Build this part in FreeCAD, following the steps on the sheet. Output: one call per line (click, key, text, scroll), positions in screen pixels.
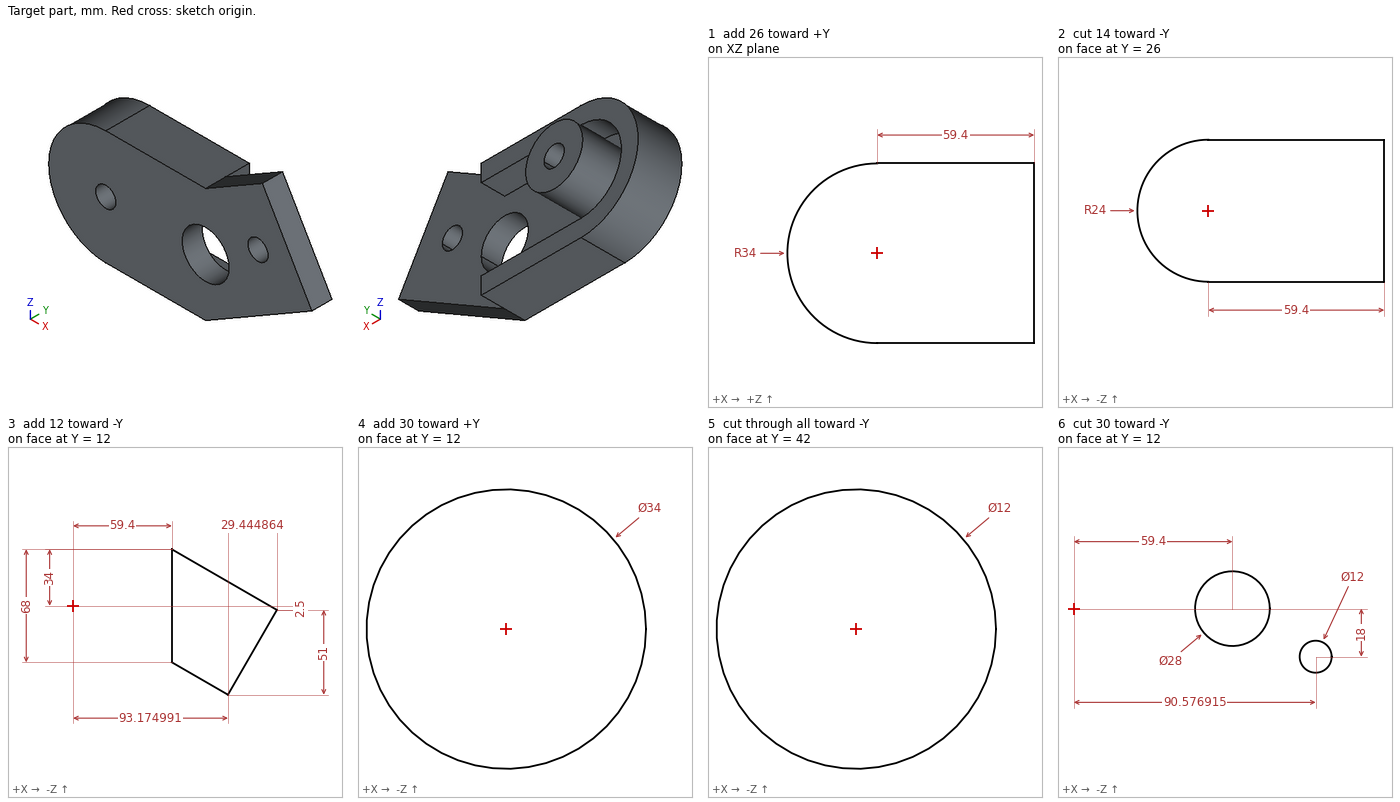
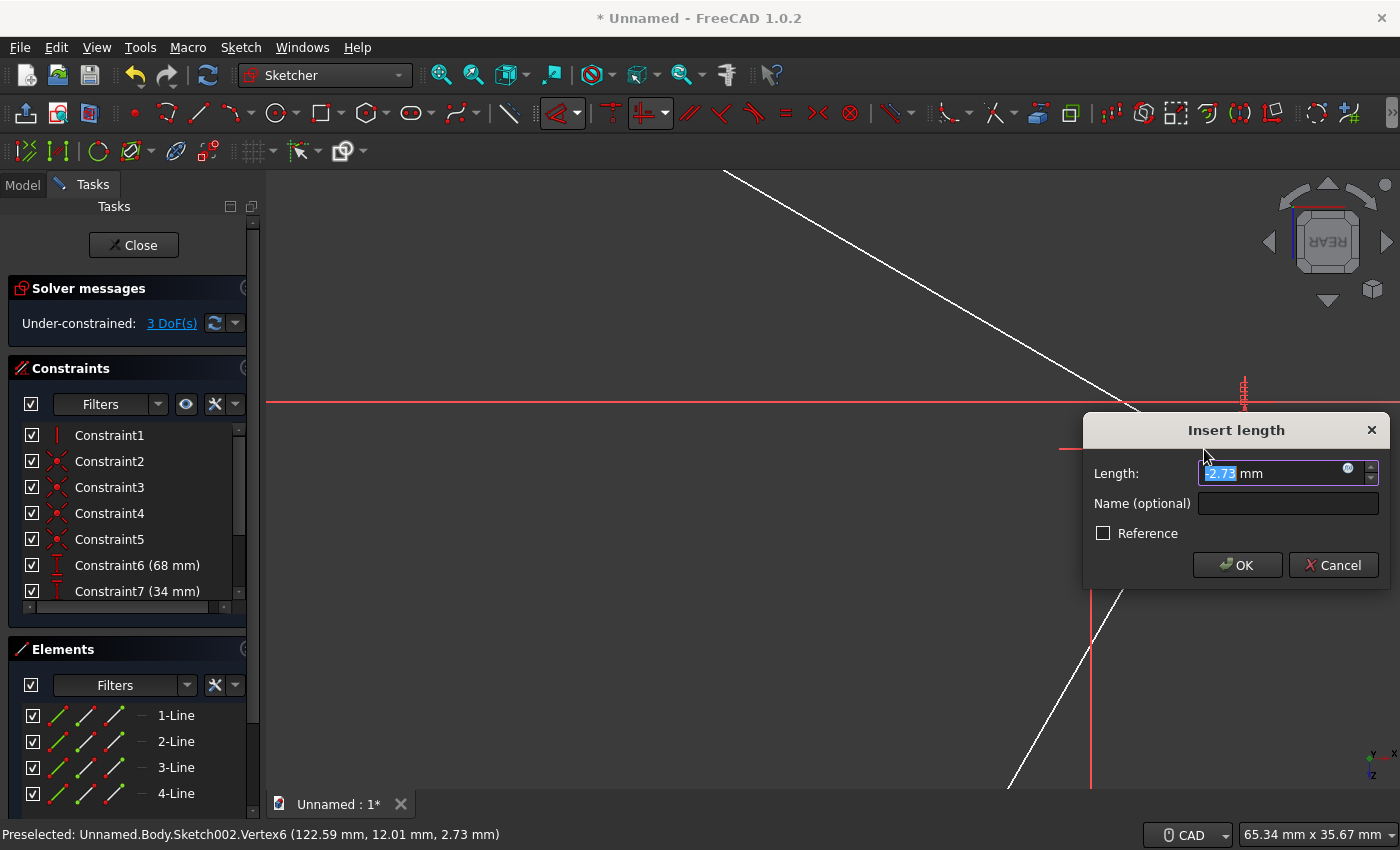
text(-2.5)
key(Return)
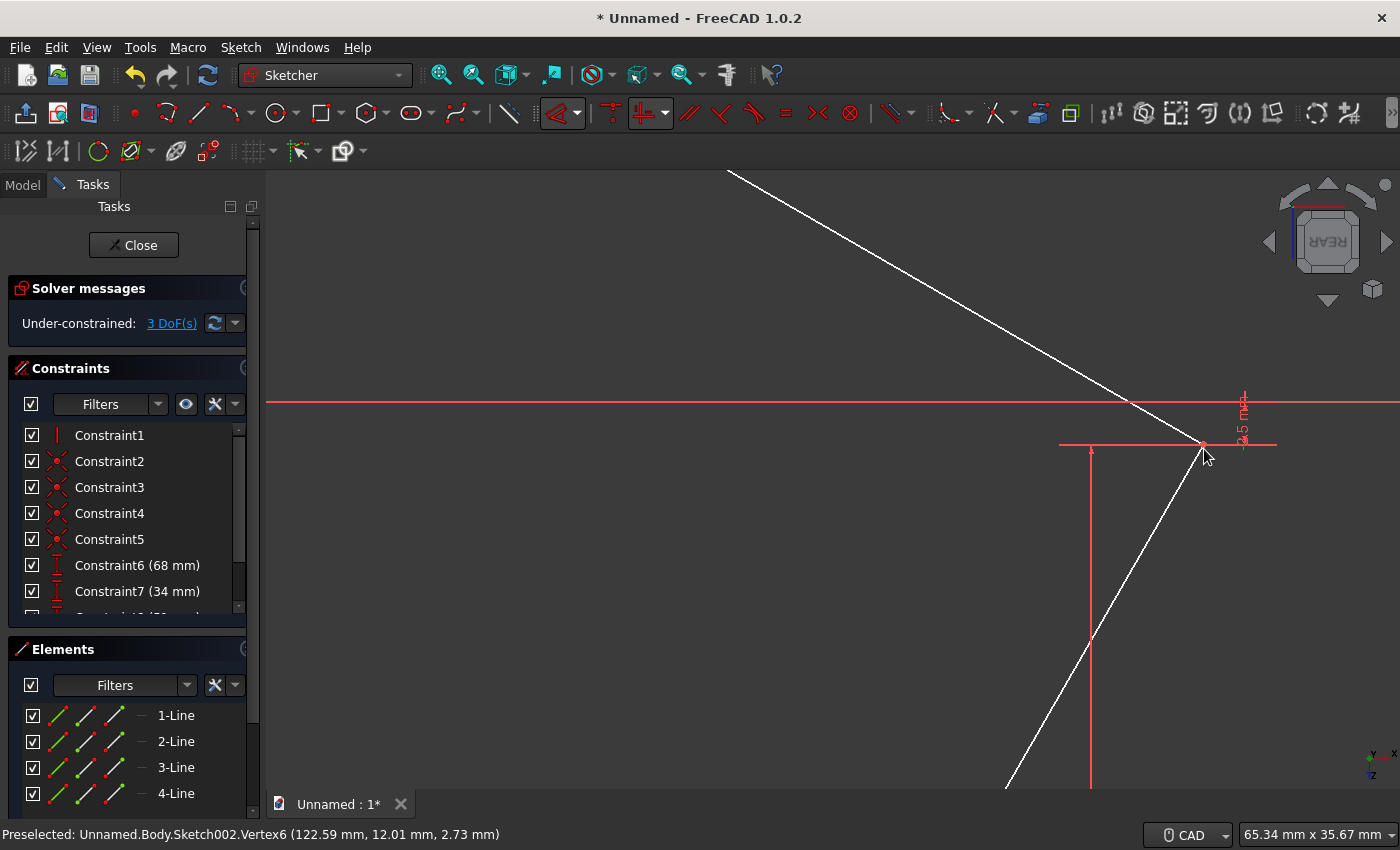
scroll(969, 450, down, 7)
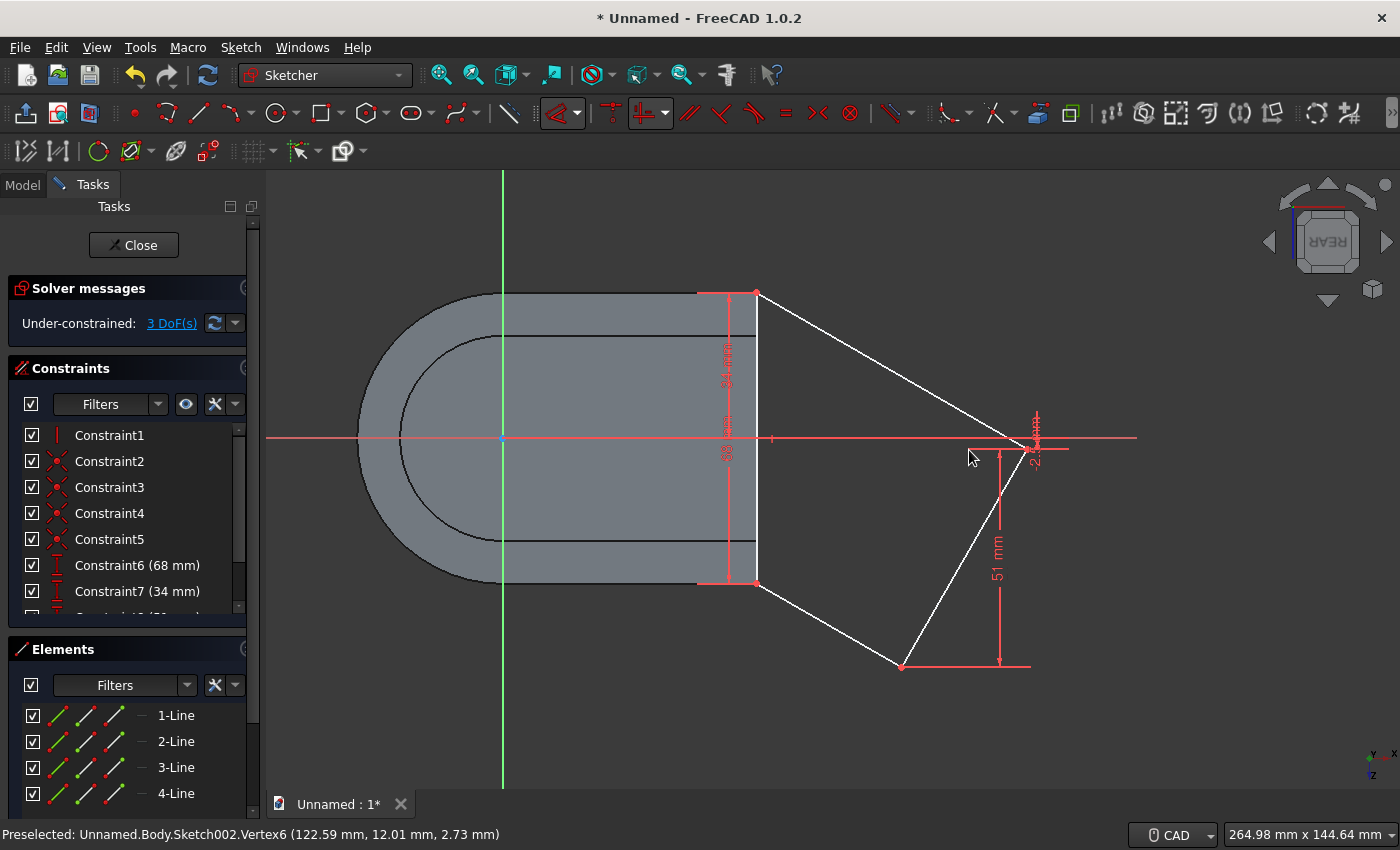
click(757, 293)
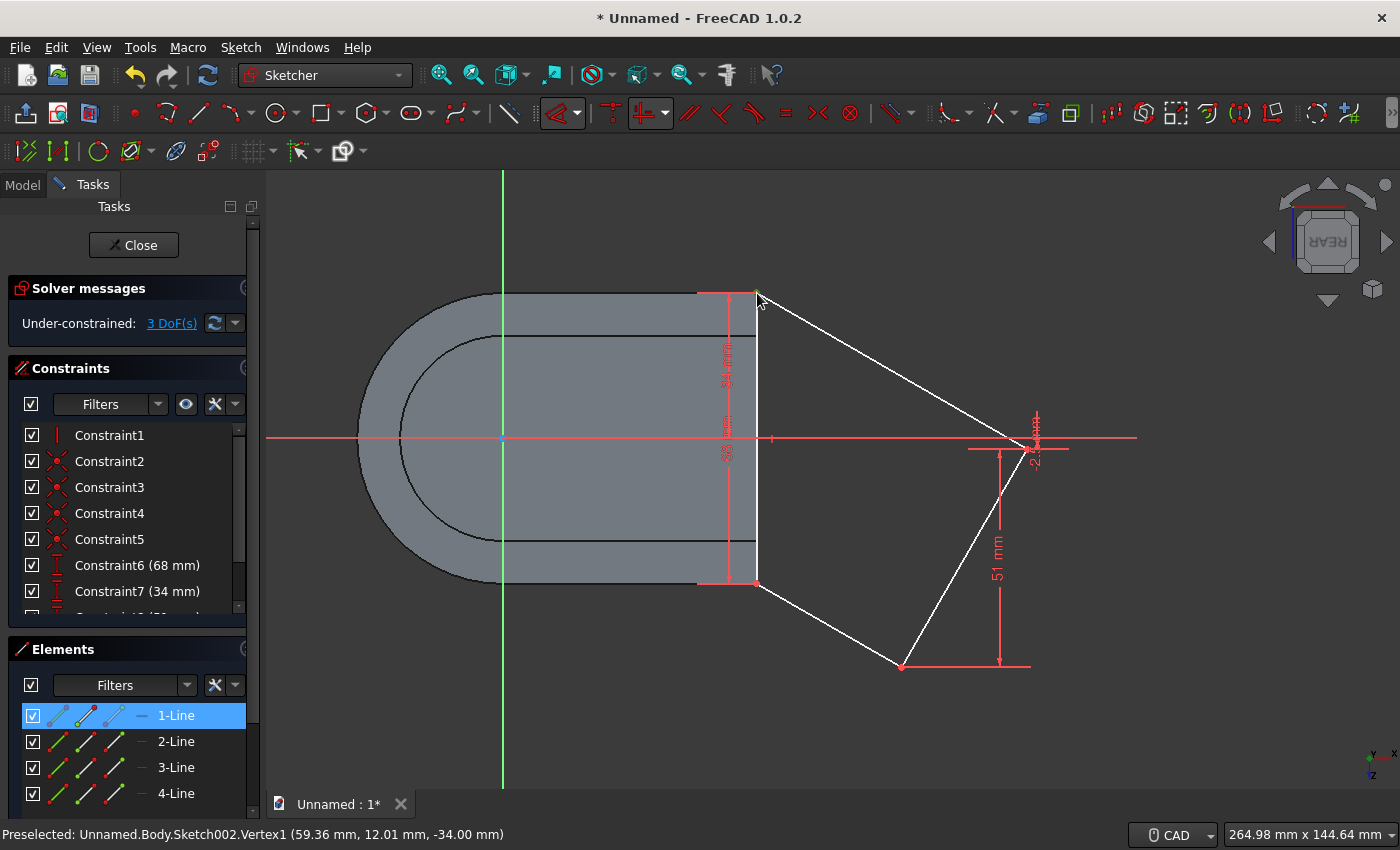
key(l)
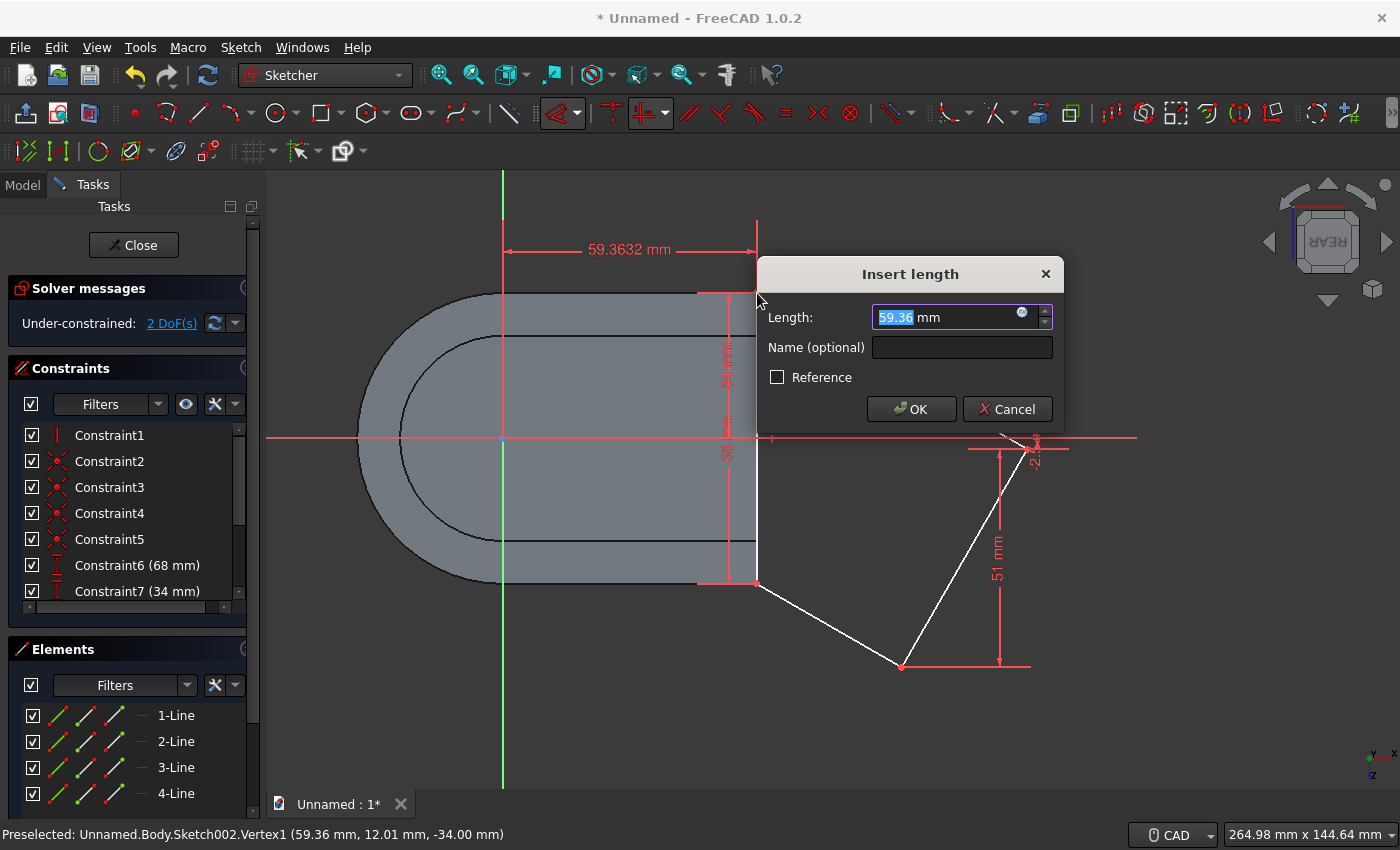
text(59.4)
key(Return)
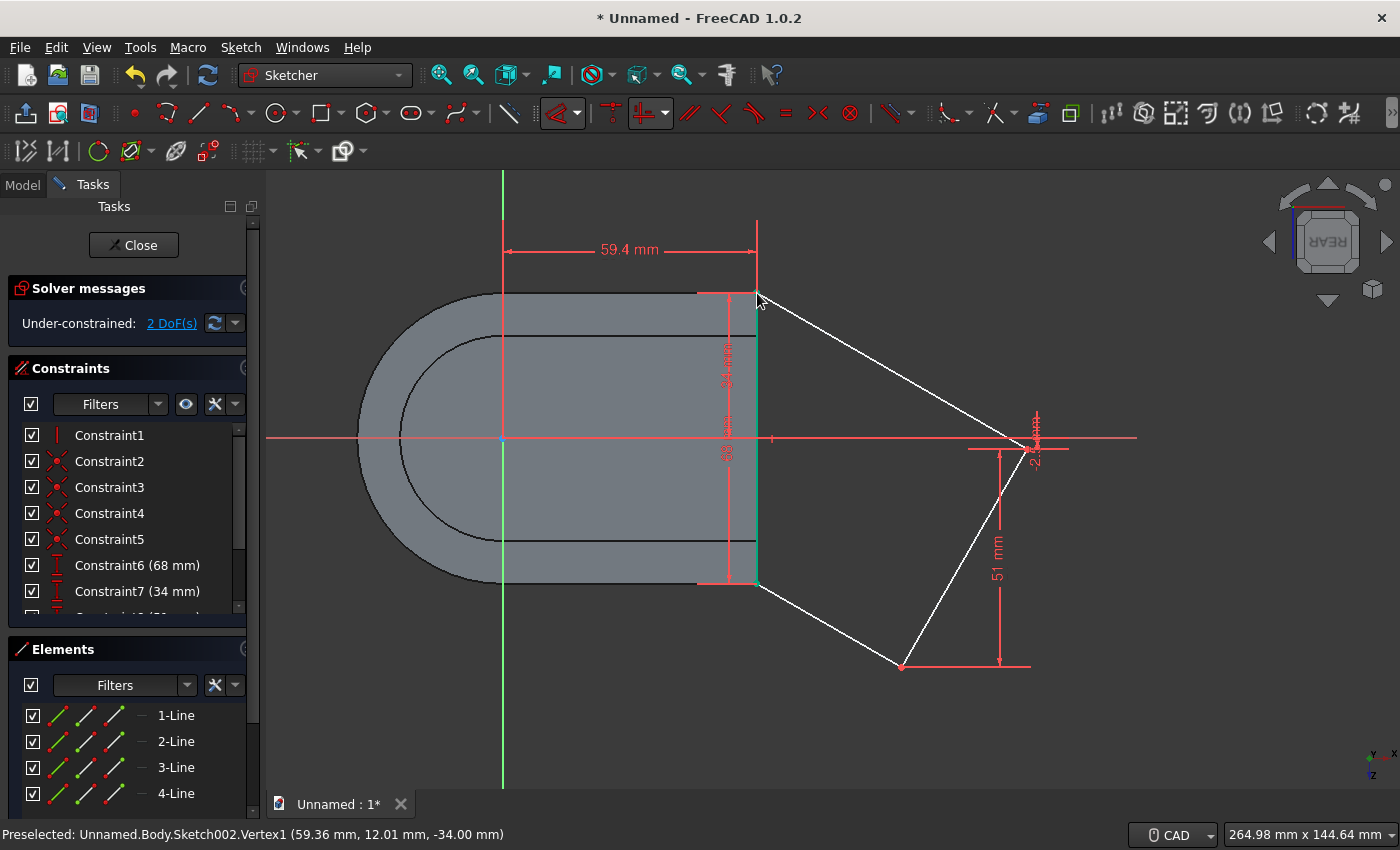
click(902, 667)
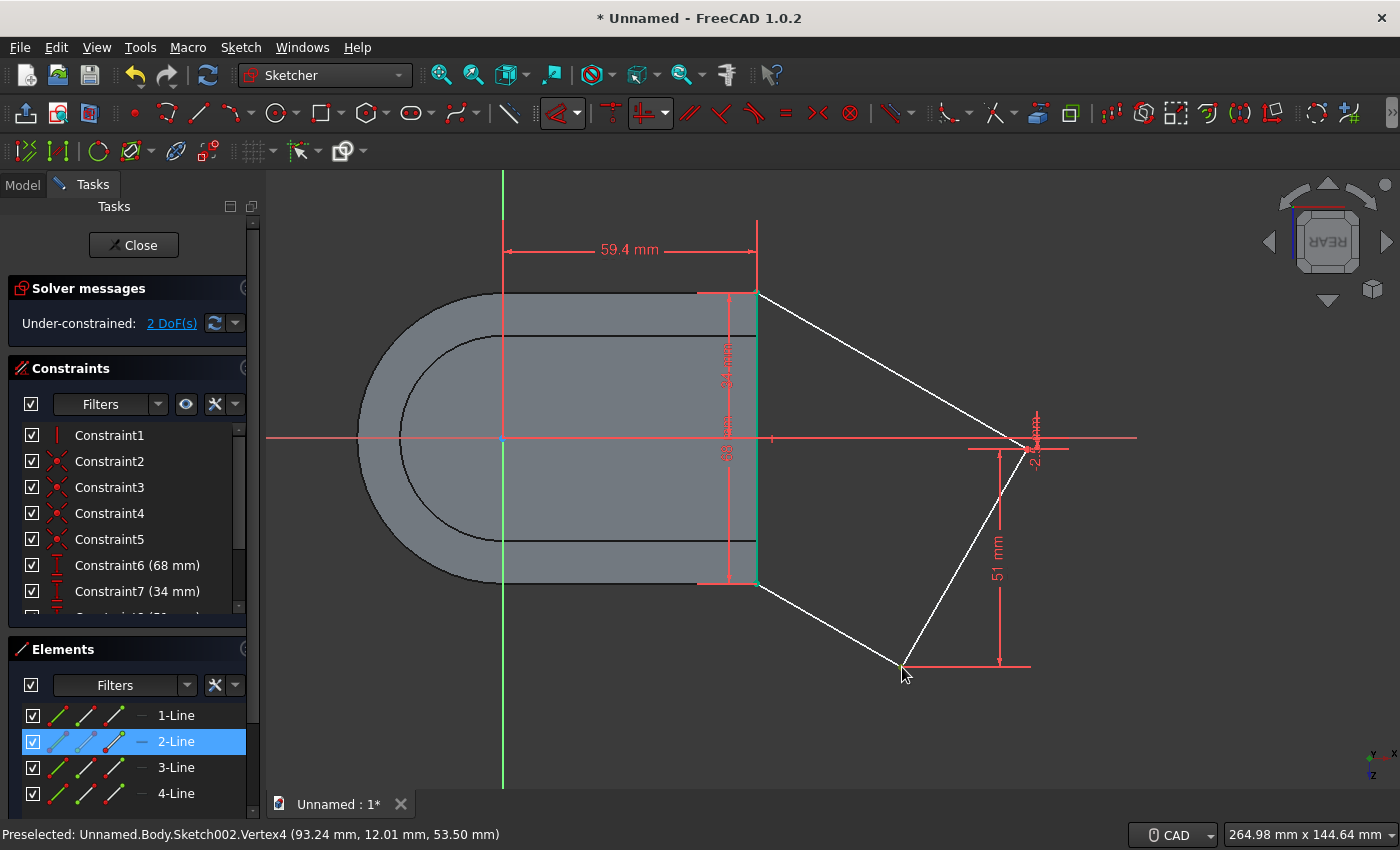
click(580, 114)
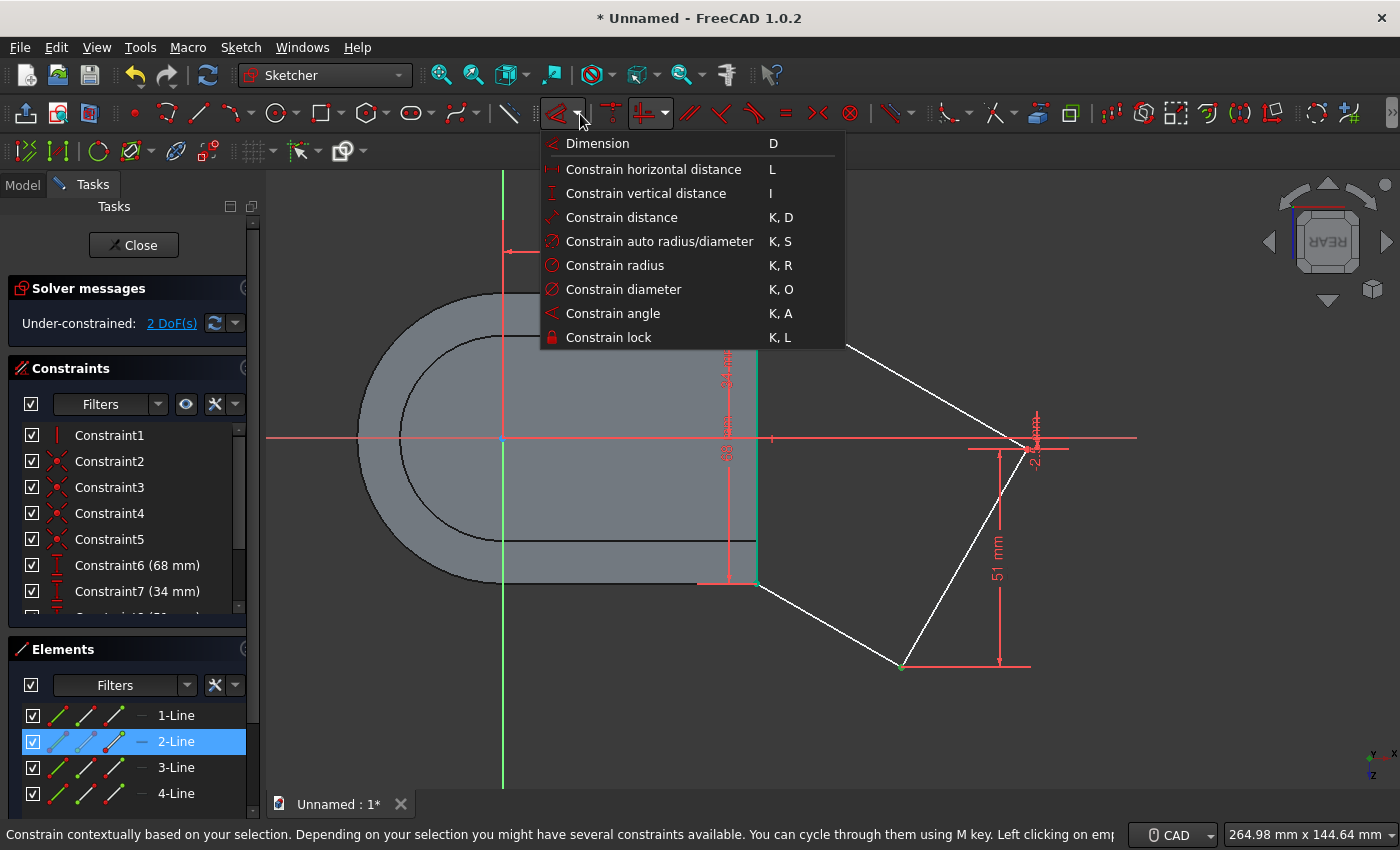
click(693, 169)